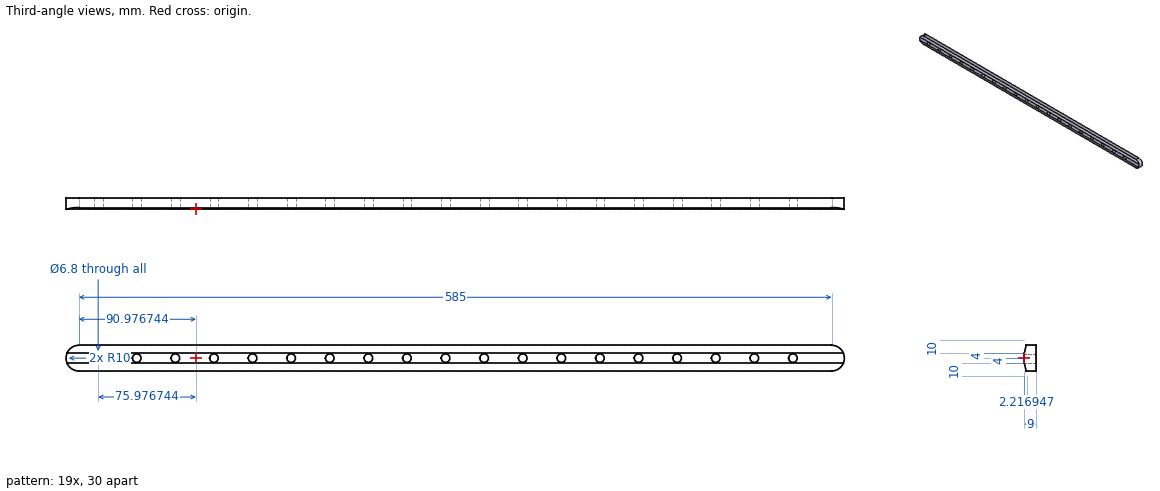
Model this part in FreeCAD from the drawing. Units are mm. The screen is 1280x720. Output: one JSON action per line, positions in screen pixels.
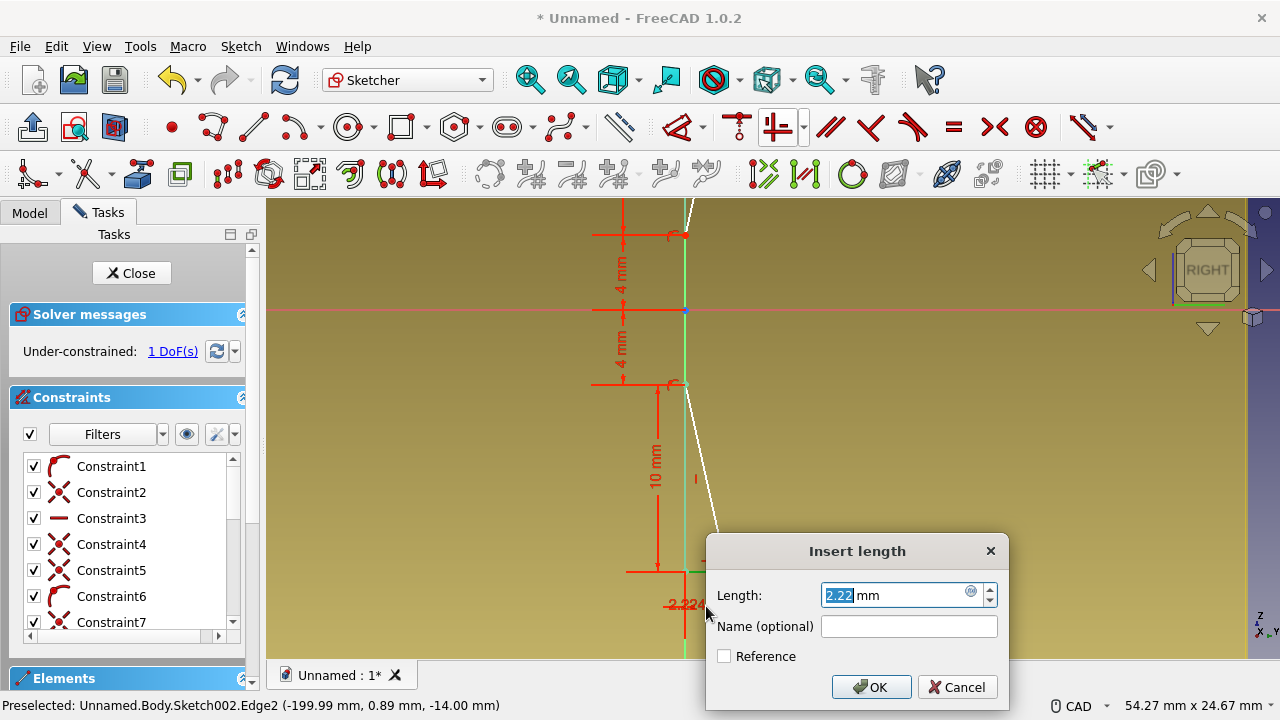
{"action": "type", "text": "2.216947"}
{"action": "key", "text": "Return"}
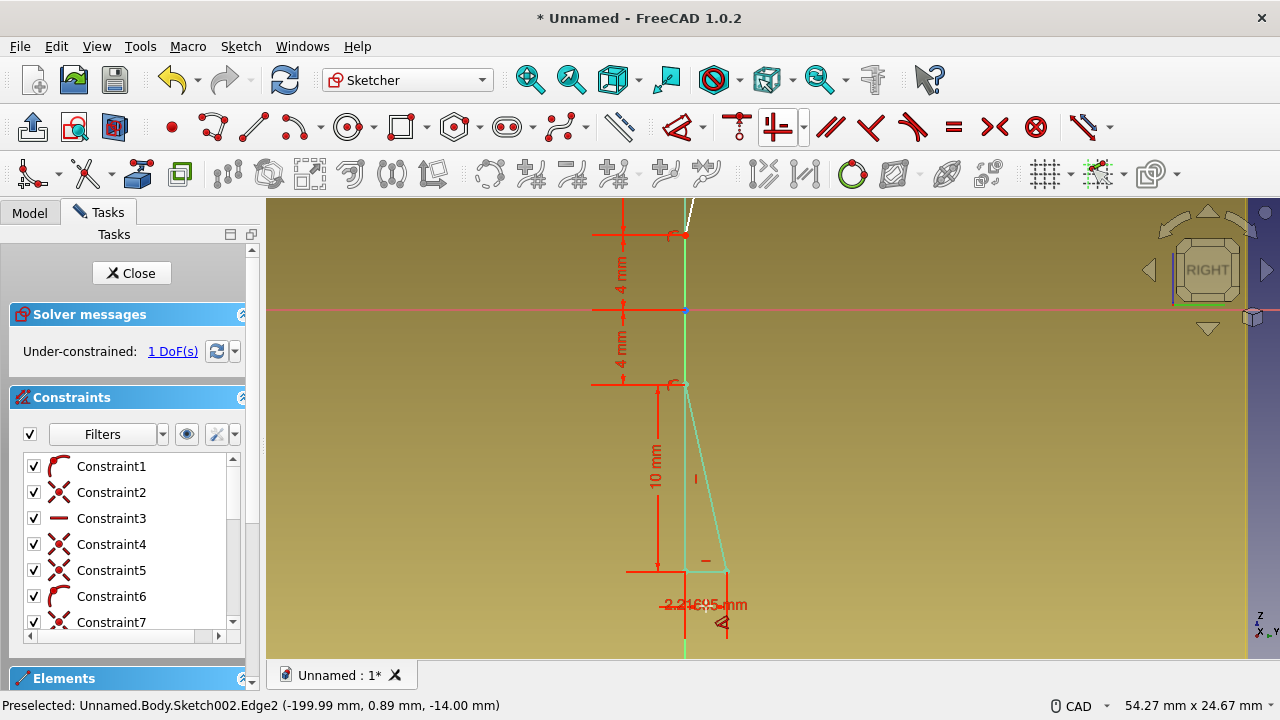
{"action": "scroll", "coordinate": [702, 572], "scroll_direction": "down", "scroll_amount": 3}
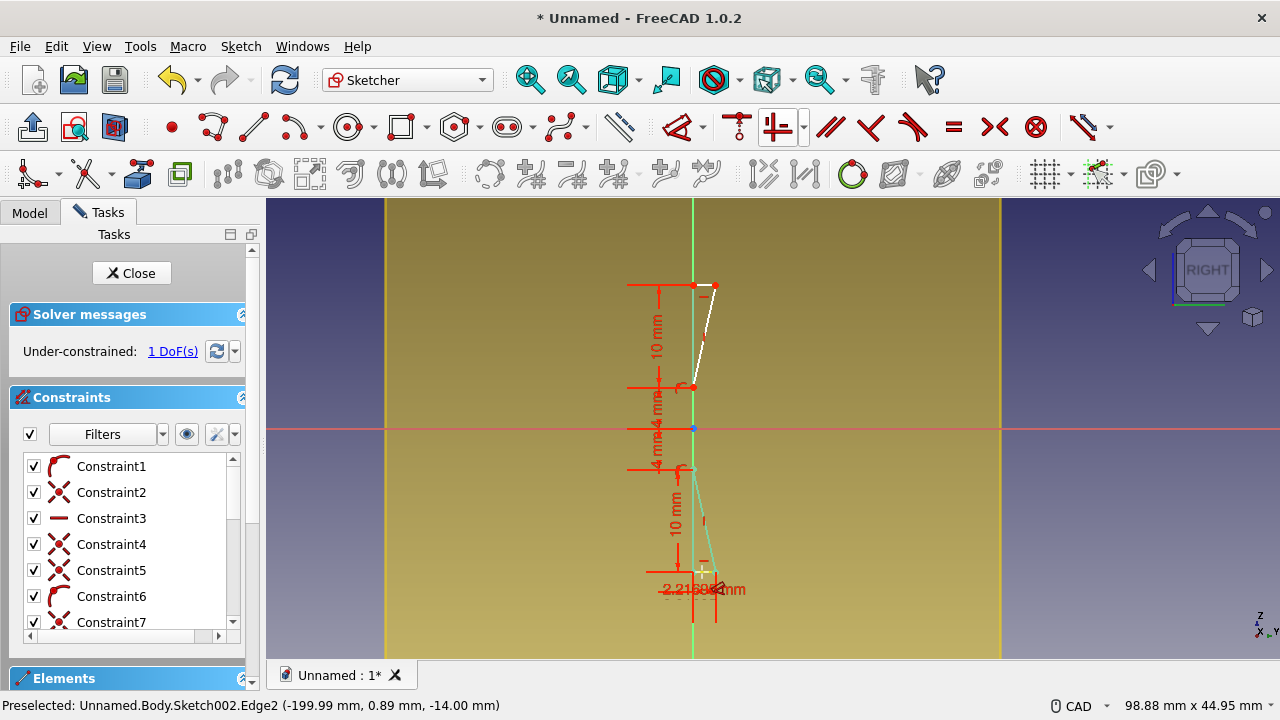
{"action": "scroll", "coordinate": [709, 285], "scroll_direction": "up", "scroll_amount": 4}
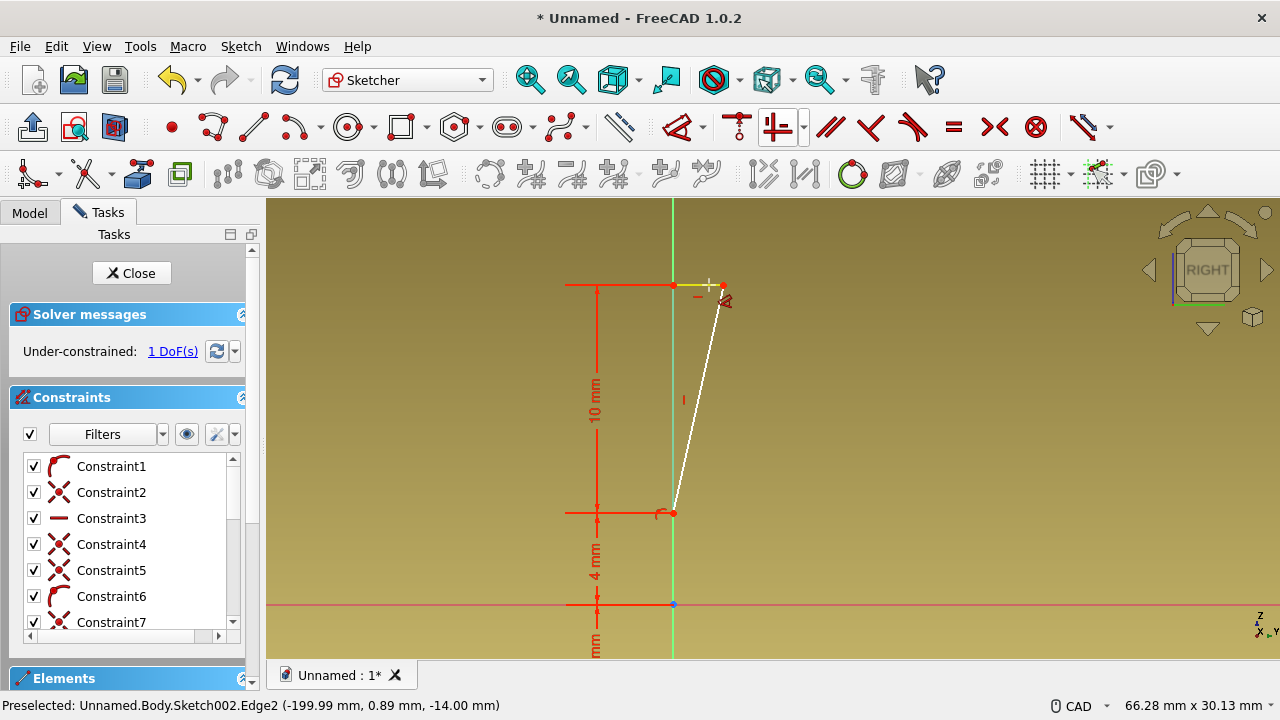
{"action": "left_click", "coordinate": [709, 285]}
{"action": "left_click", "coordinate": [698, 251]}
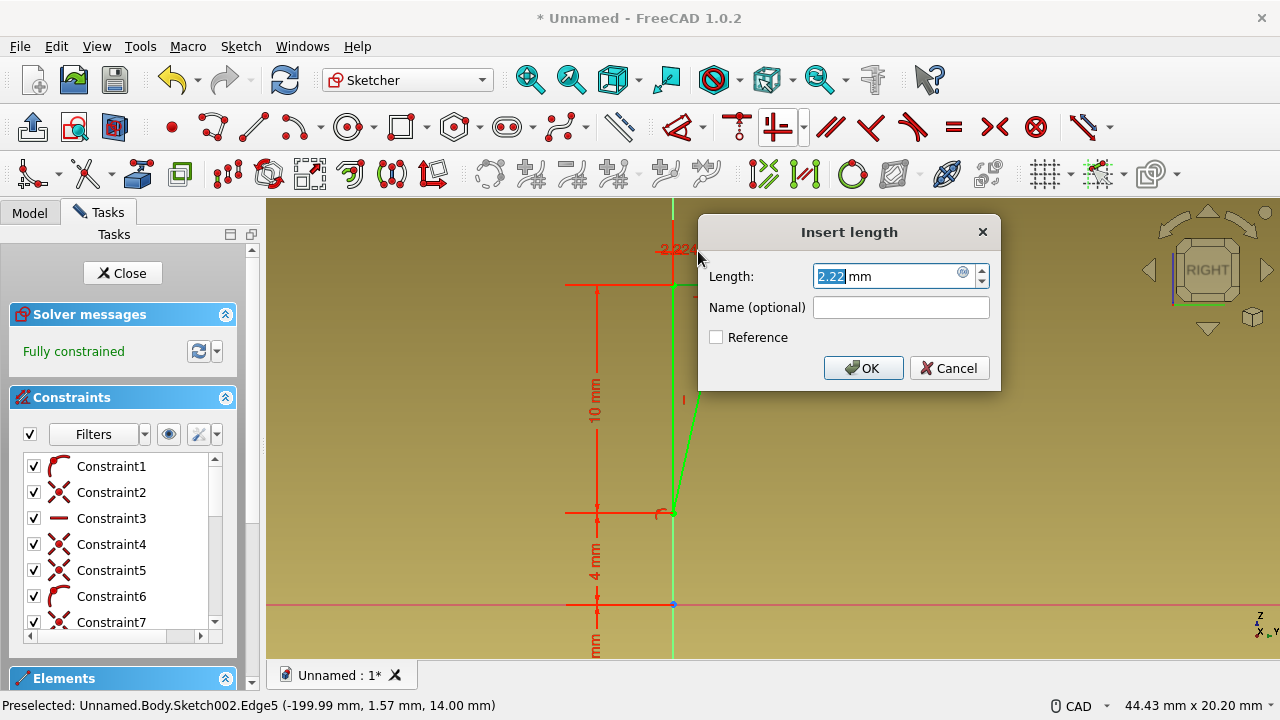
{"action": "type", "text": "2.216947"}
{"action": "key", "text": "Return"}
{"action": "key", "text": "Escape"}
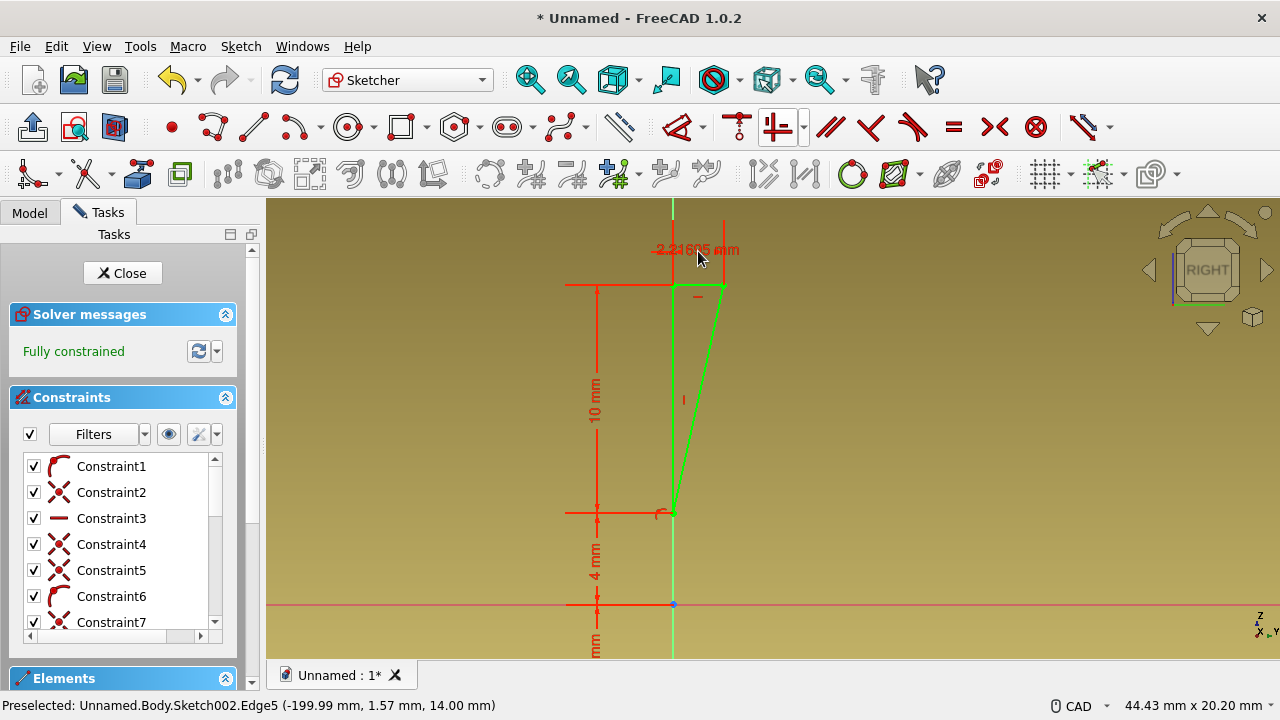
{"action": "left_click", "coordinate": [123, 273]}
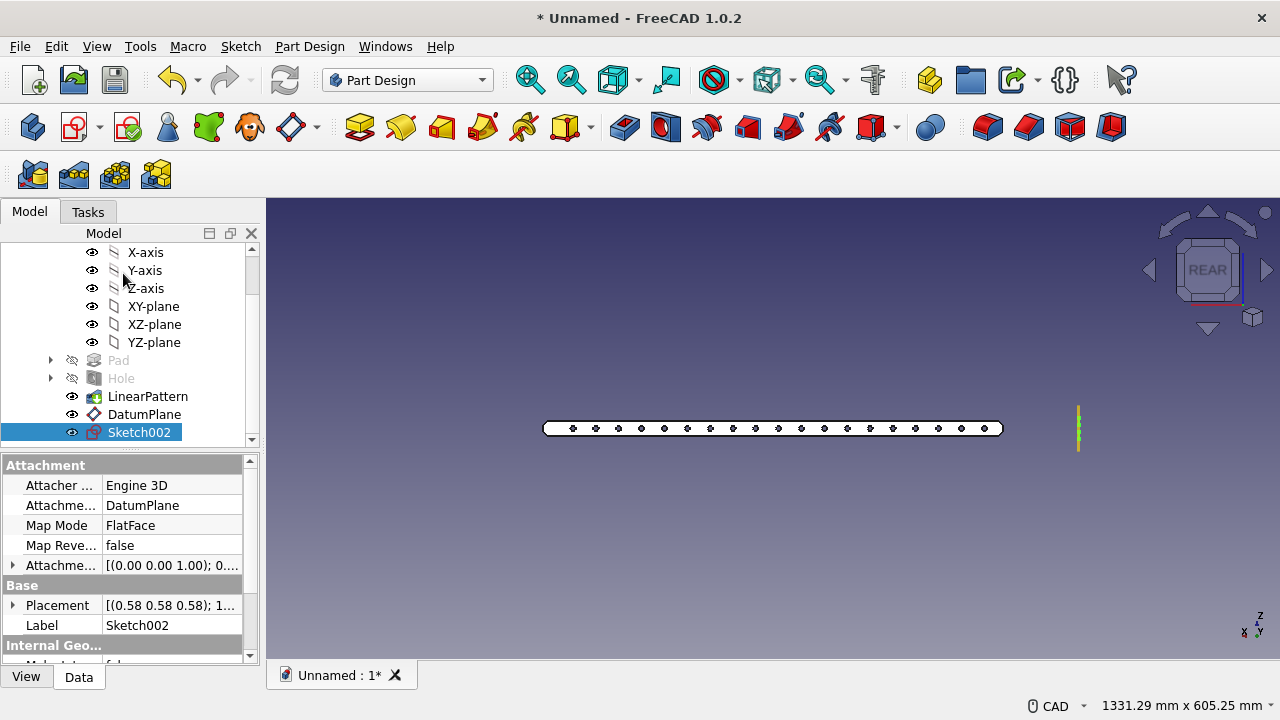
{"action": "left_click", "coordinate": [625, 128]}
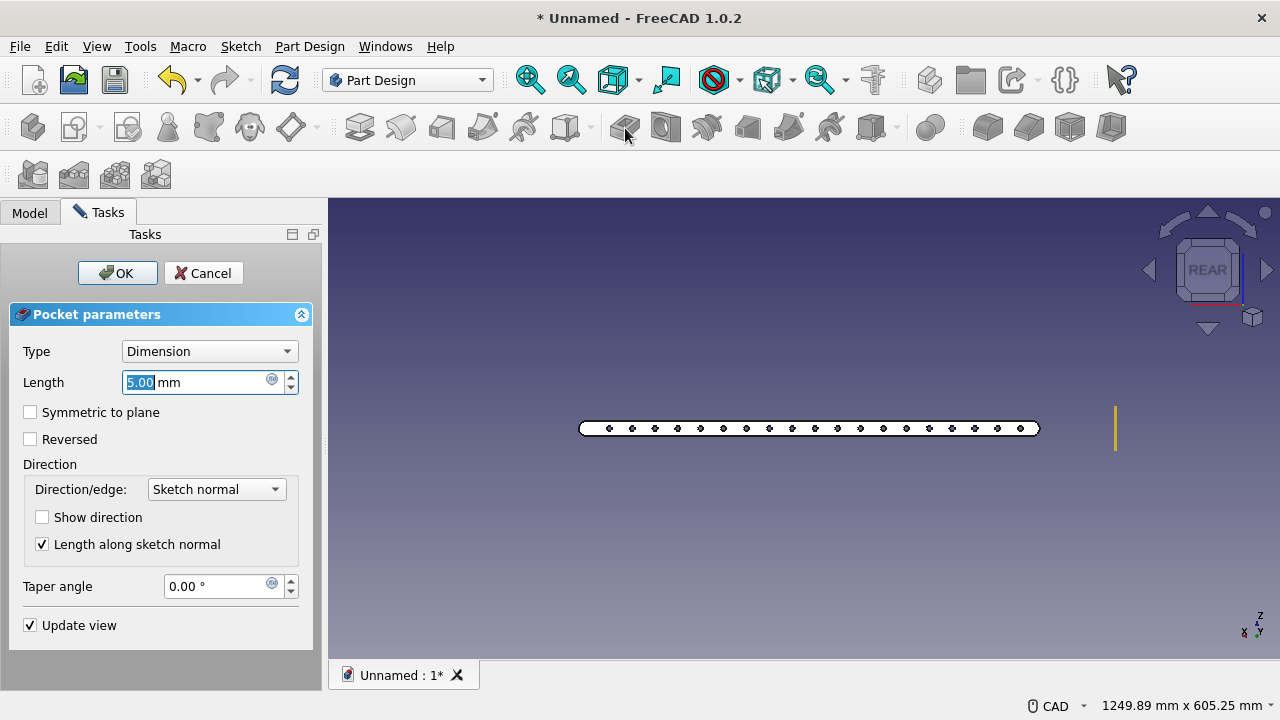
{"action": "left_click", "coordinate": [210, 352]}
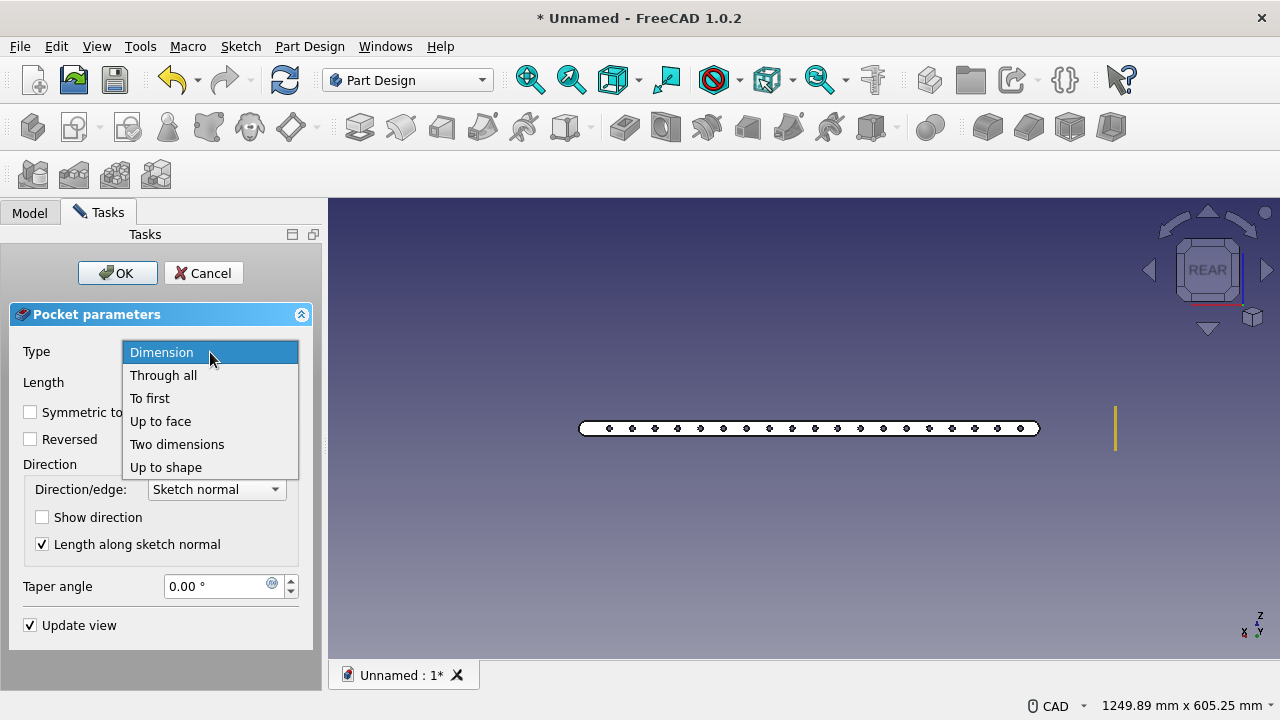
{"action": "left_click", "coordinate": [208, 376]}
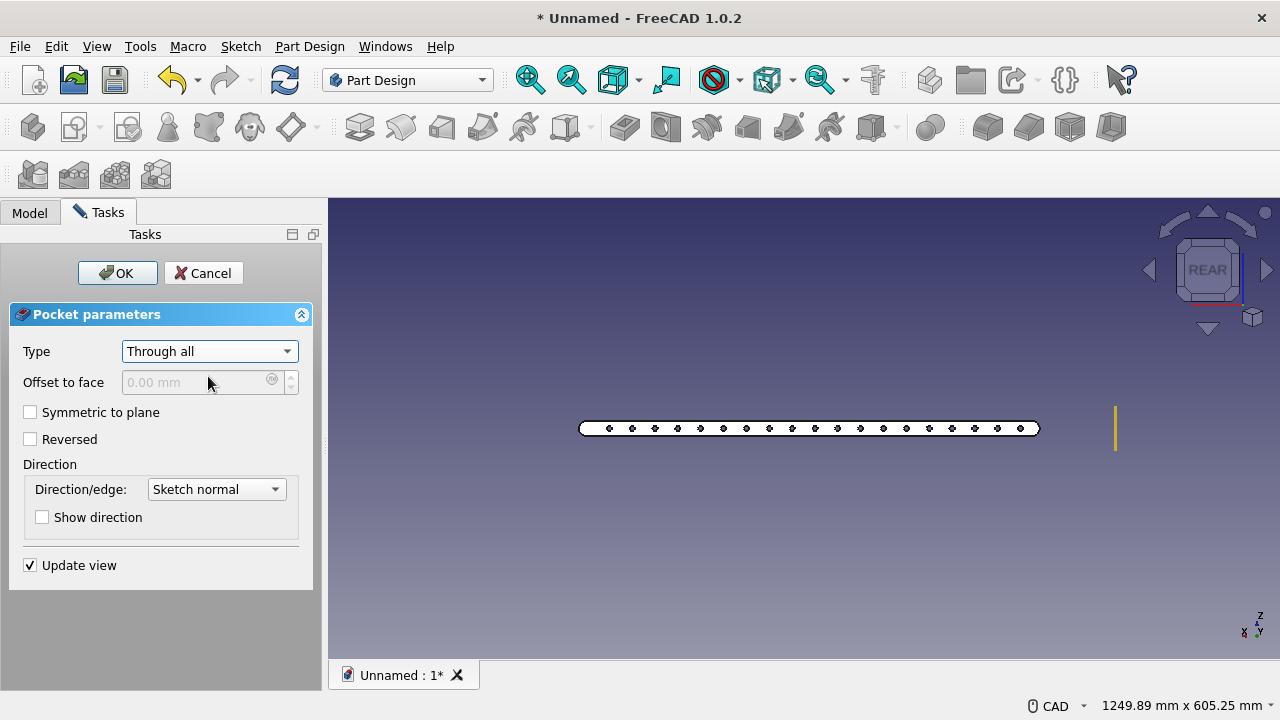
{"action": "left_click", "coordinate": [31, 439]}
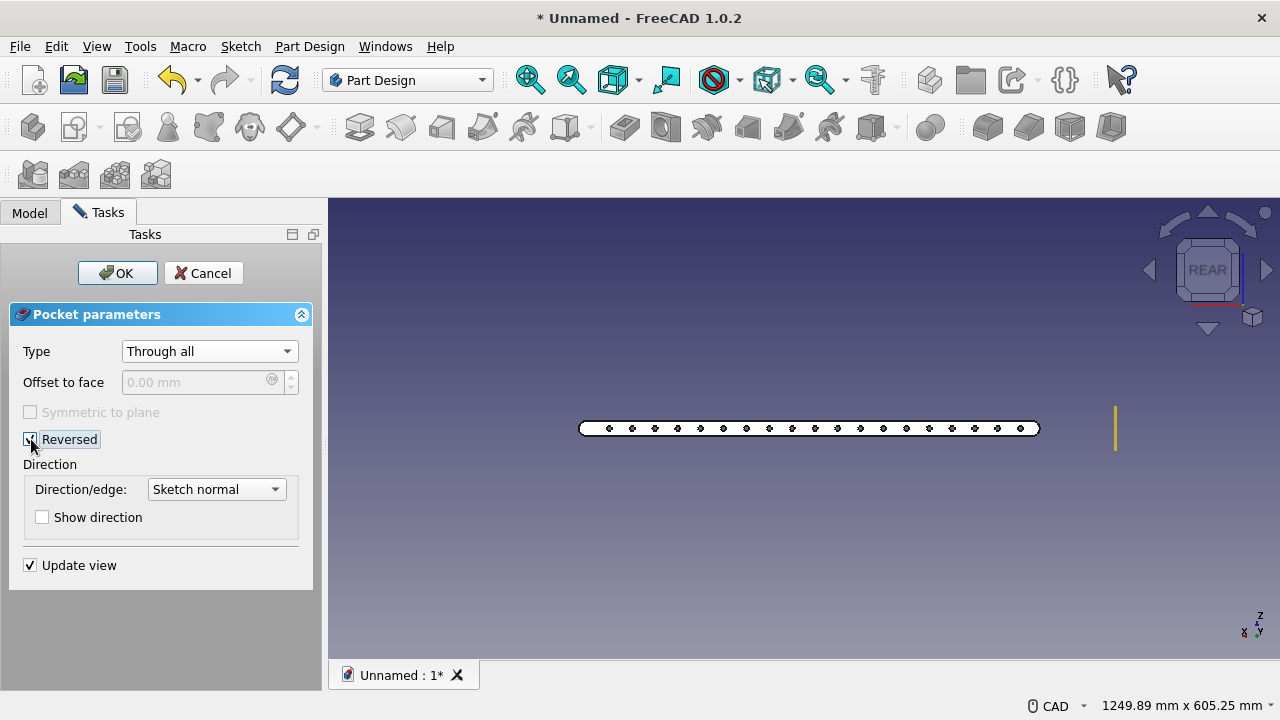
{"action": "left_click", "coordinate": [118, 273]}